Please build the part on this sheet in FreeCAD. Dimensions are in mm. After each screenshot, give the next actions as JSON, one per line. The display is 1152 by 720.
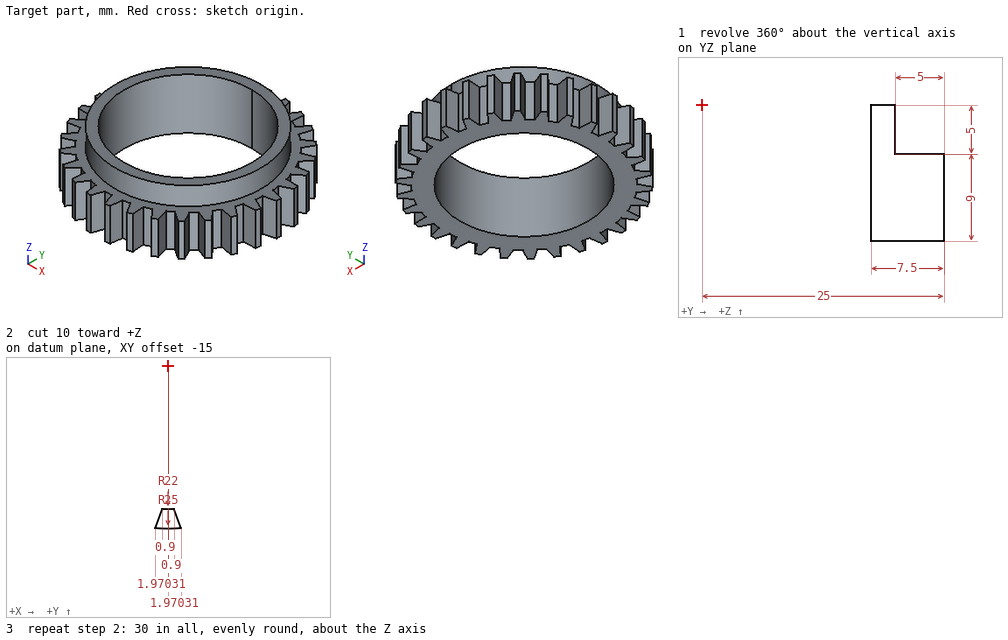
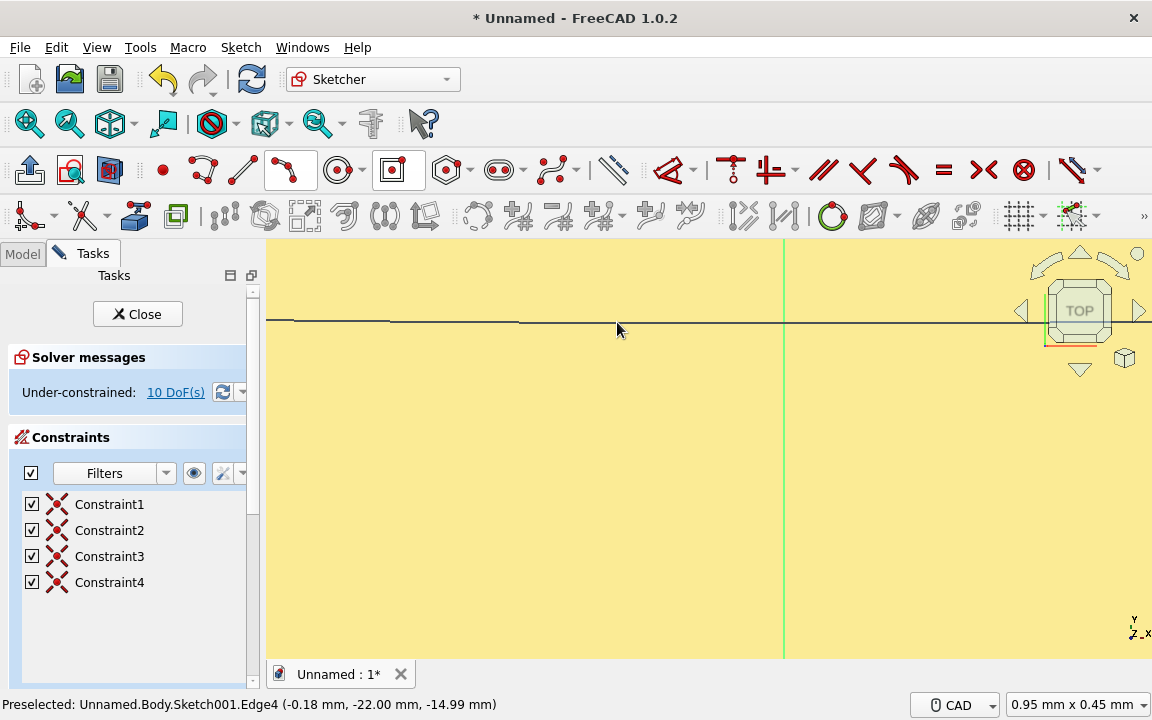
{"action": "scroll", "coordinate": [626, 323], "scroll_direction": "down", "scroll_amount": 12}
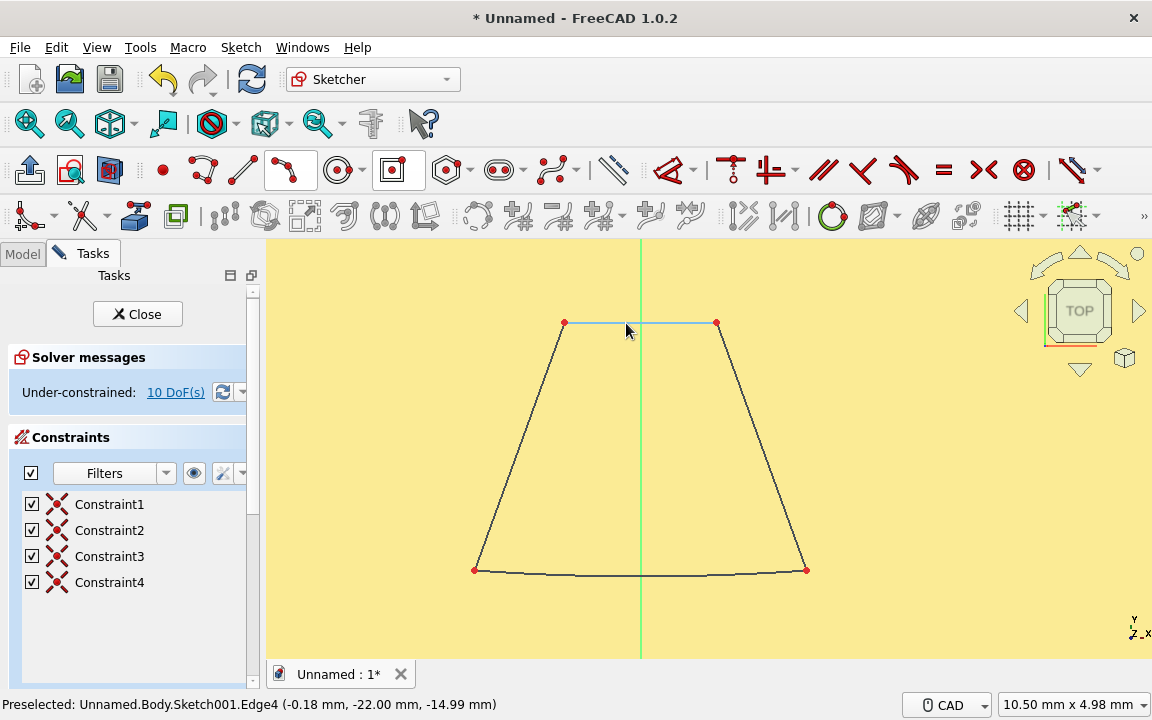
{"action": "left_click", "coordinate": [574, 575]}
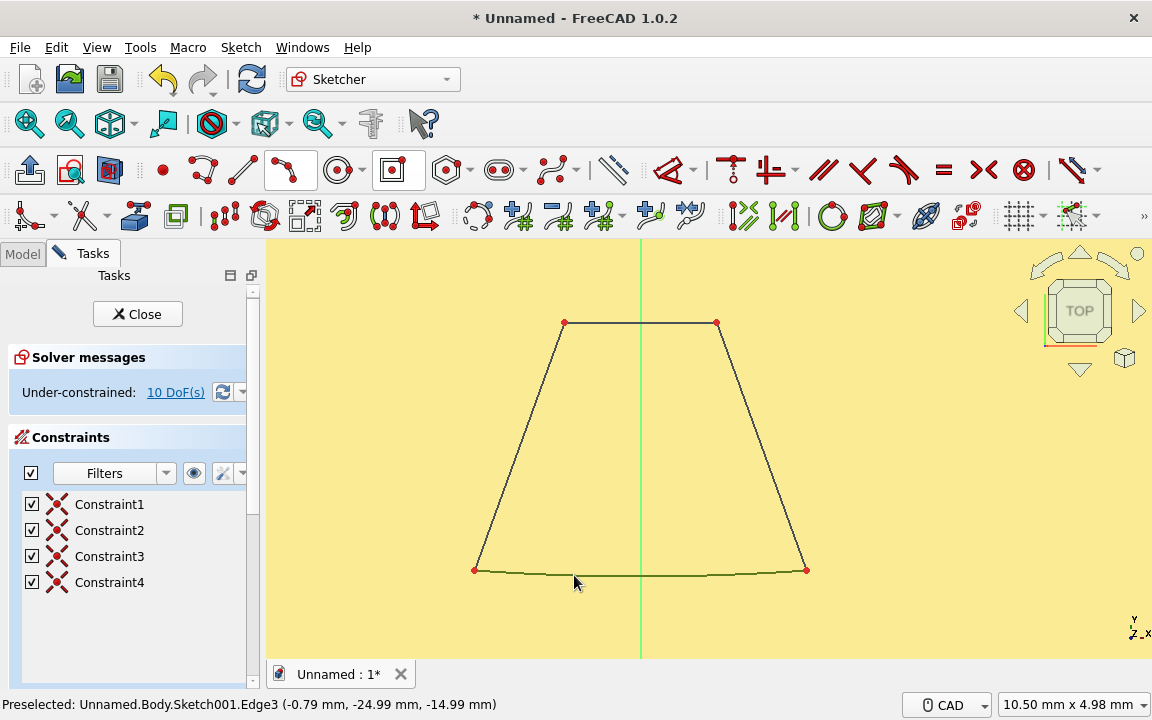
{"action": "left_click", "coordinate": [610, 323]}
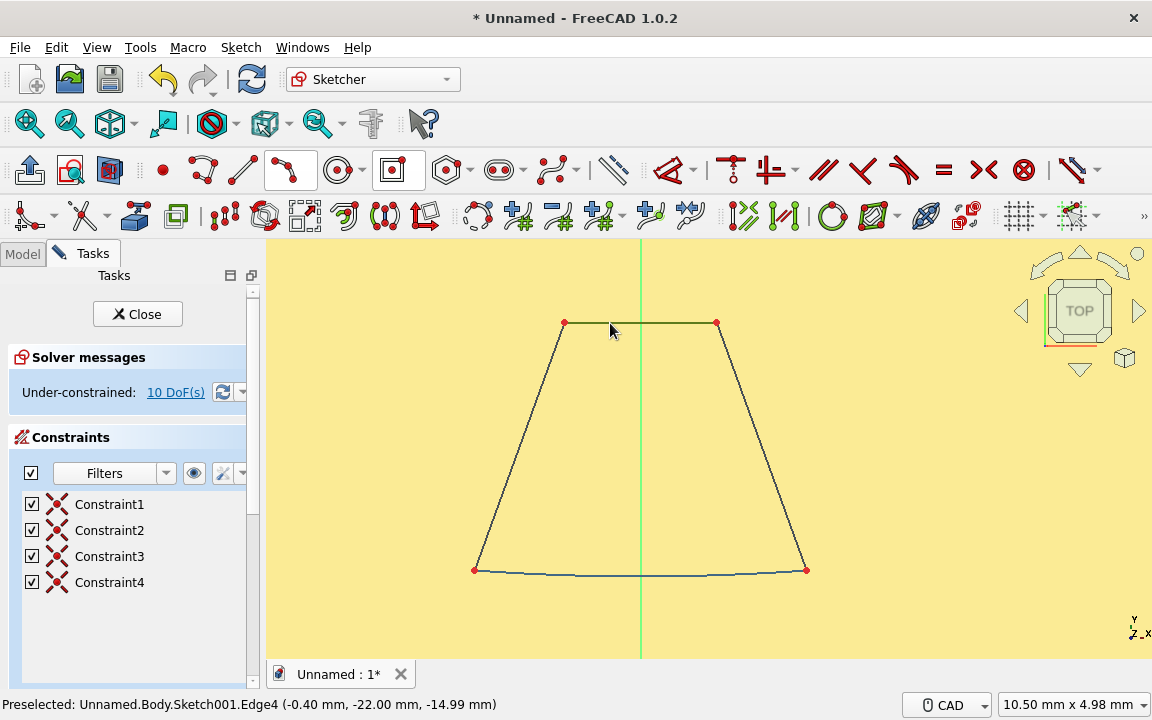
{"action": "left_click", "coordinate": [732, 170]}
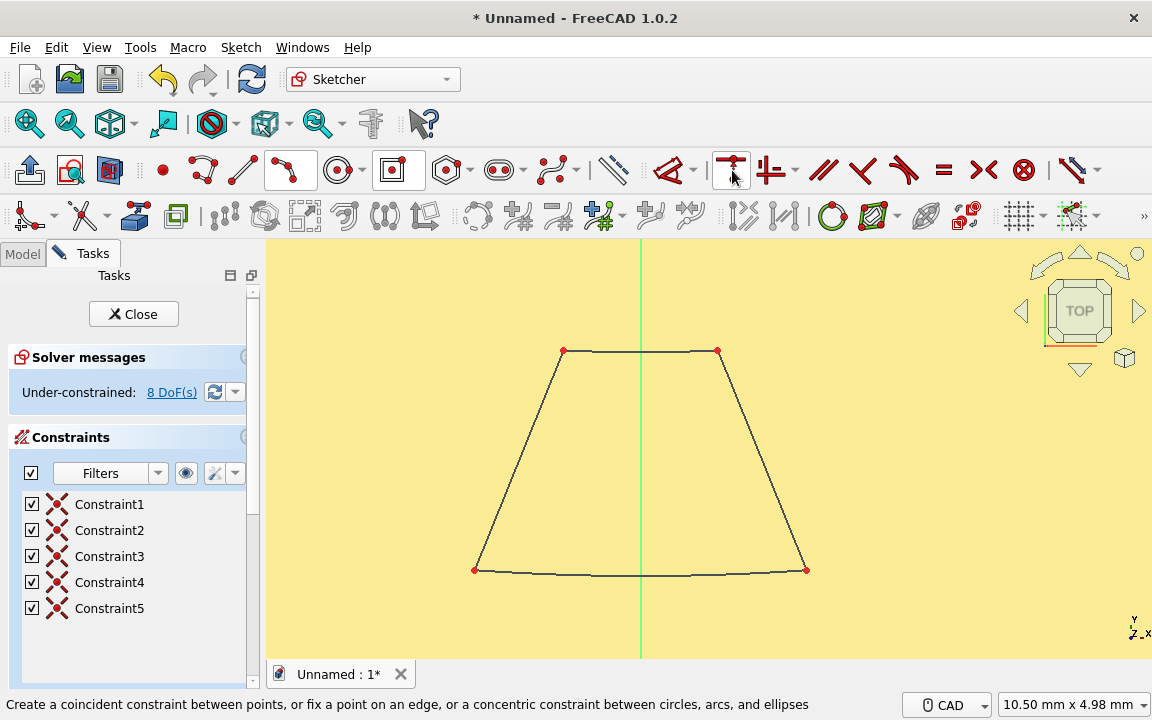
{"action": "scroll", "coordinate": [640, 572], "scroll_direction": "down", "scroll_amount": 11}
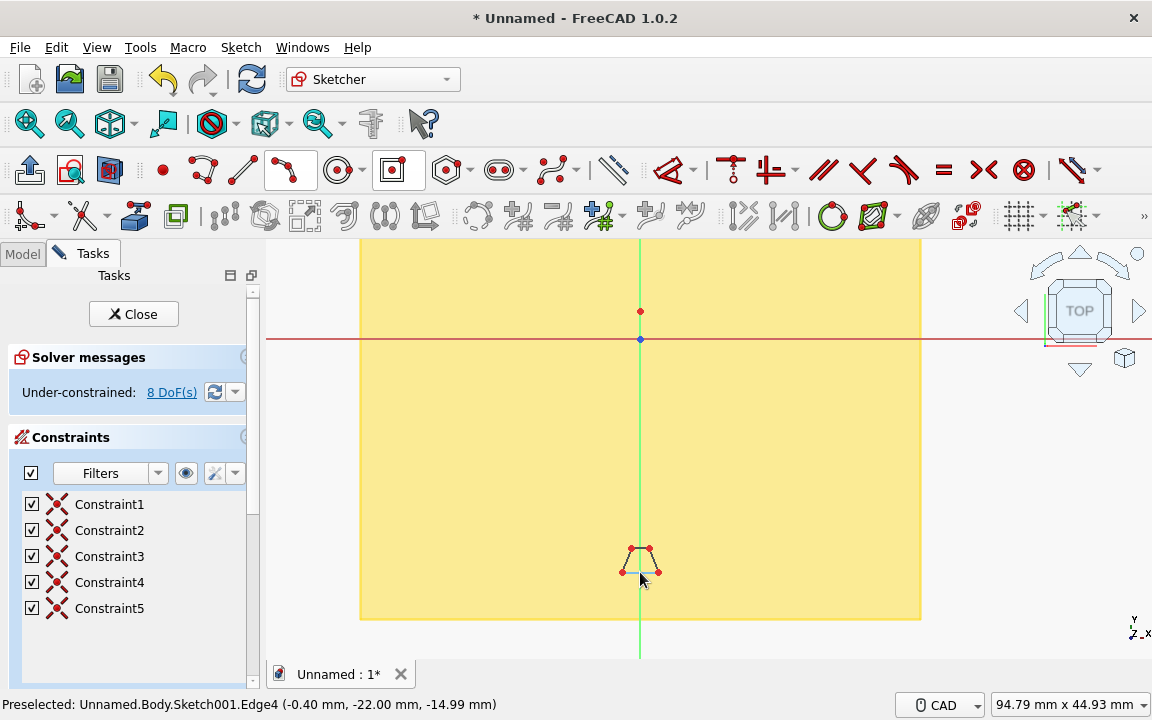
{"action": "left_click_drag", "start_coordinate": [630, 302], "coordinate": [650, 349]}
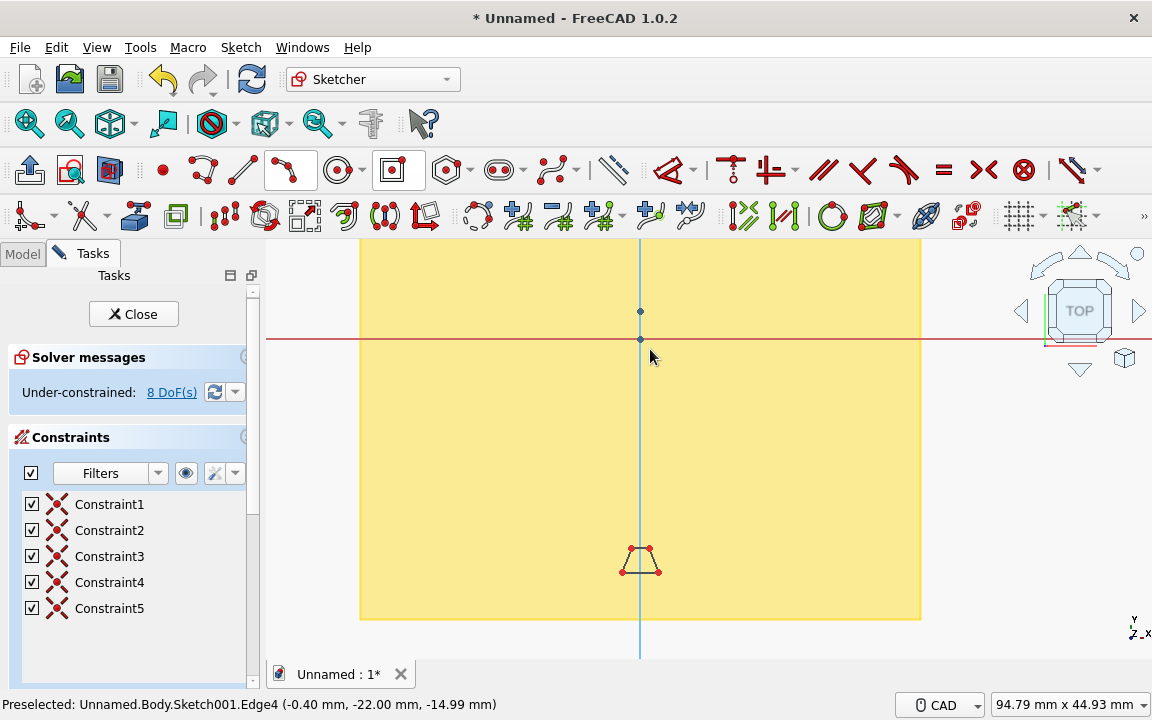
{"action": "left_click", "coordinate": [732, 170]}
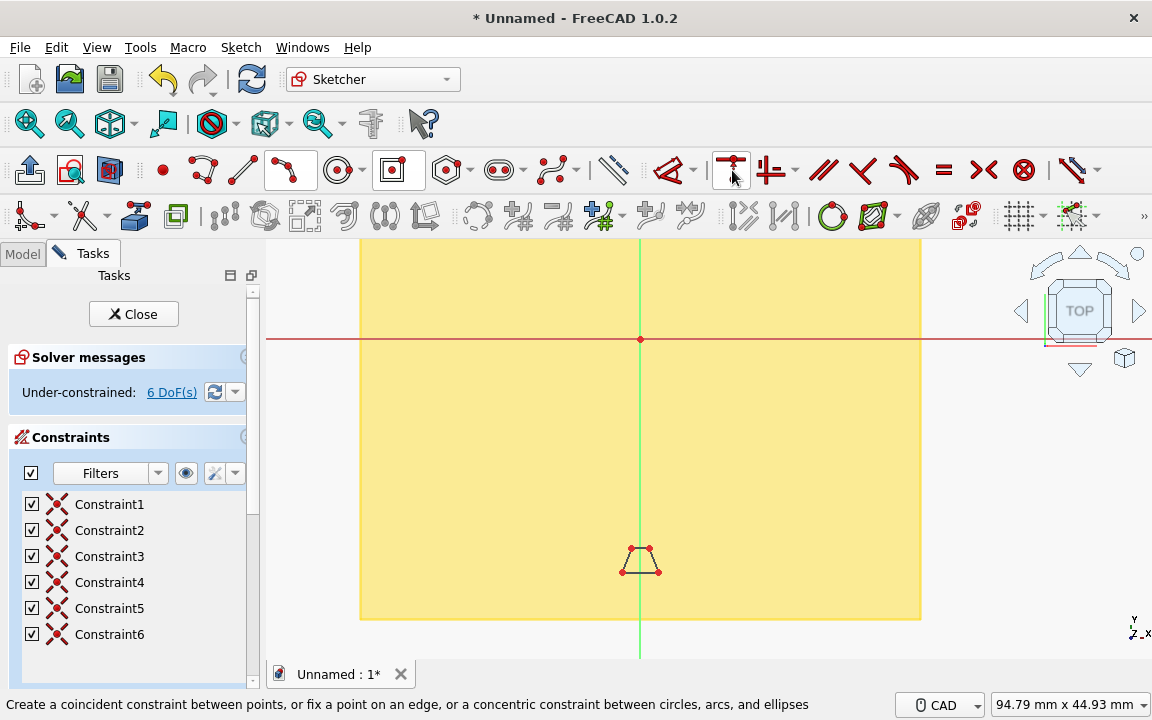
{"action": "left_click", "coordinate": [668, 170]}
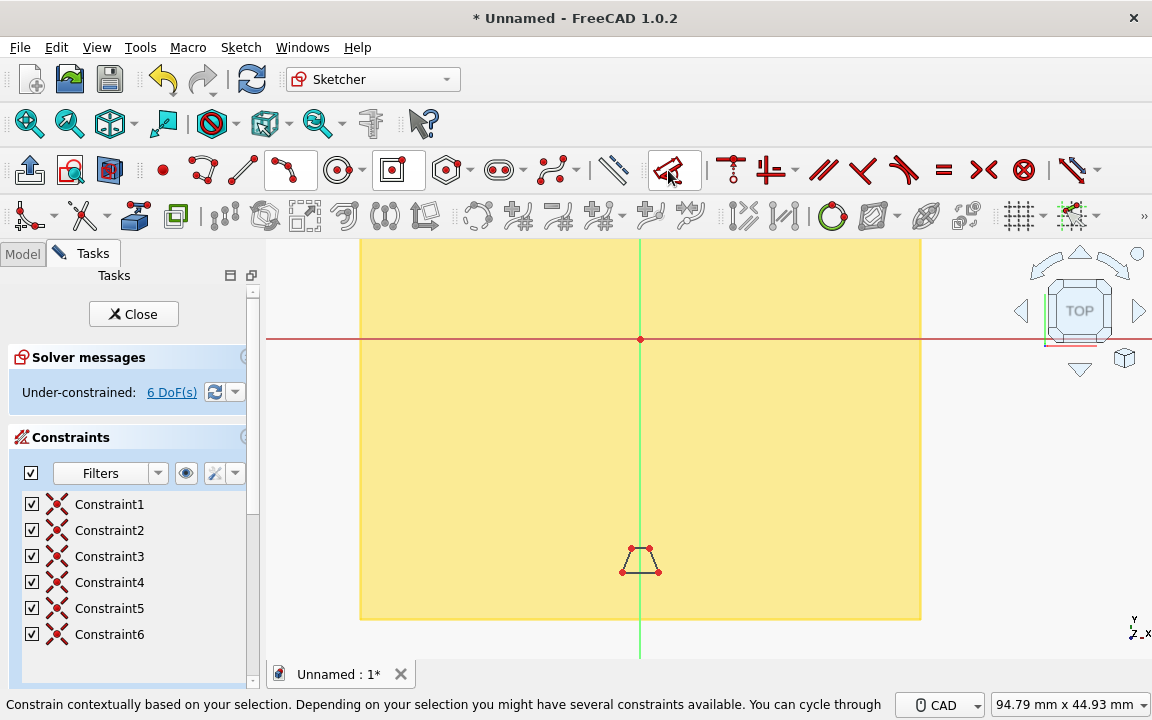
{"action": "left_click", "coordinate": [640, 573]}
{"action": "left_click", "coordinate": [513, 572]}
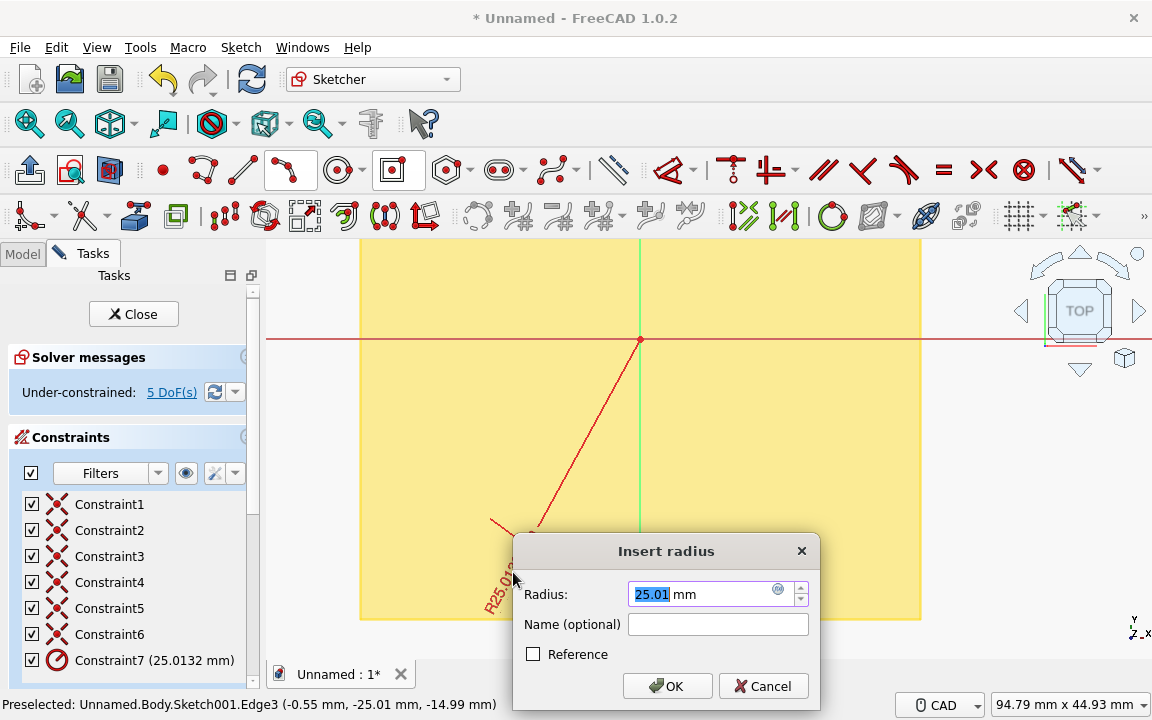
{"action": "type", "text": "25"}
{"action": "key", "text": "Return"}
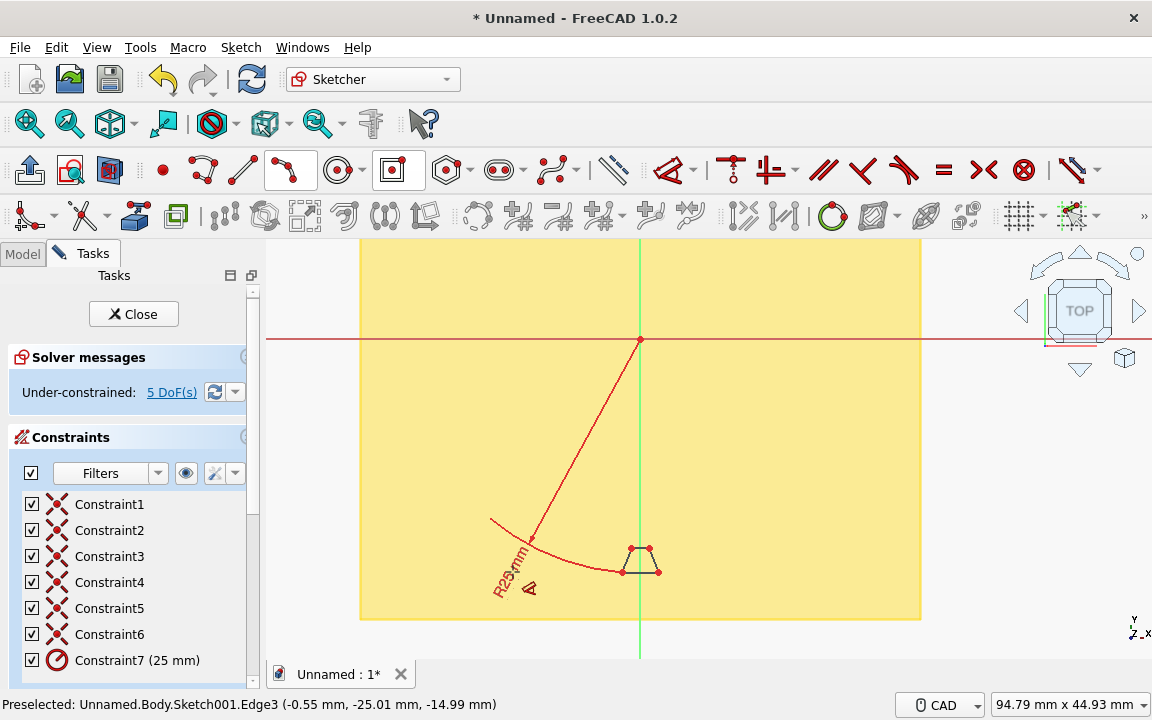
{"action": "scroll", "coordinate": [640, 548], "scroll_direction": "up", "scroll_amount": 3}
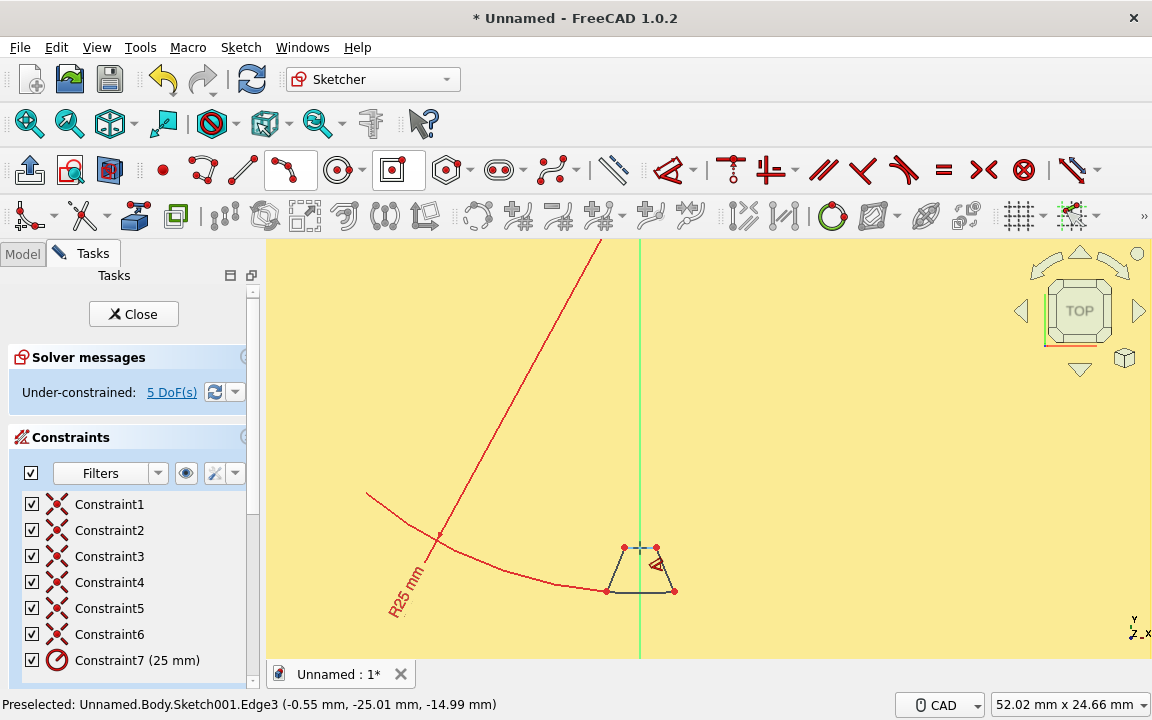
{"action": "left_click", "coordinate": [640, 548]}
{"action": "left_click", "coordinate": [442, 529]}